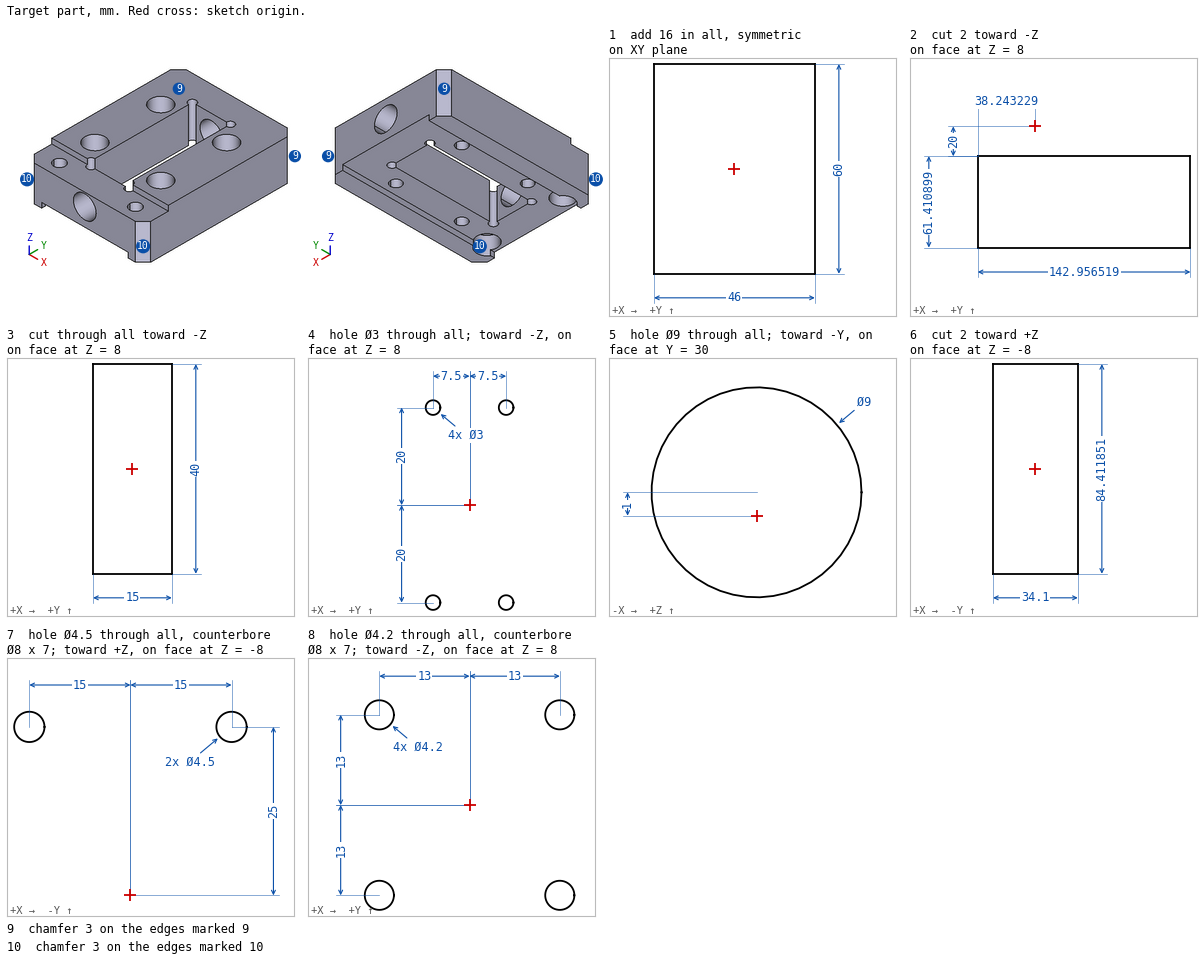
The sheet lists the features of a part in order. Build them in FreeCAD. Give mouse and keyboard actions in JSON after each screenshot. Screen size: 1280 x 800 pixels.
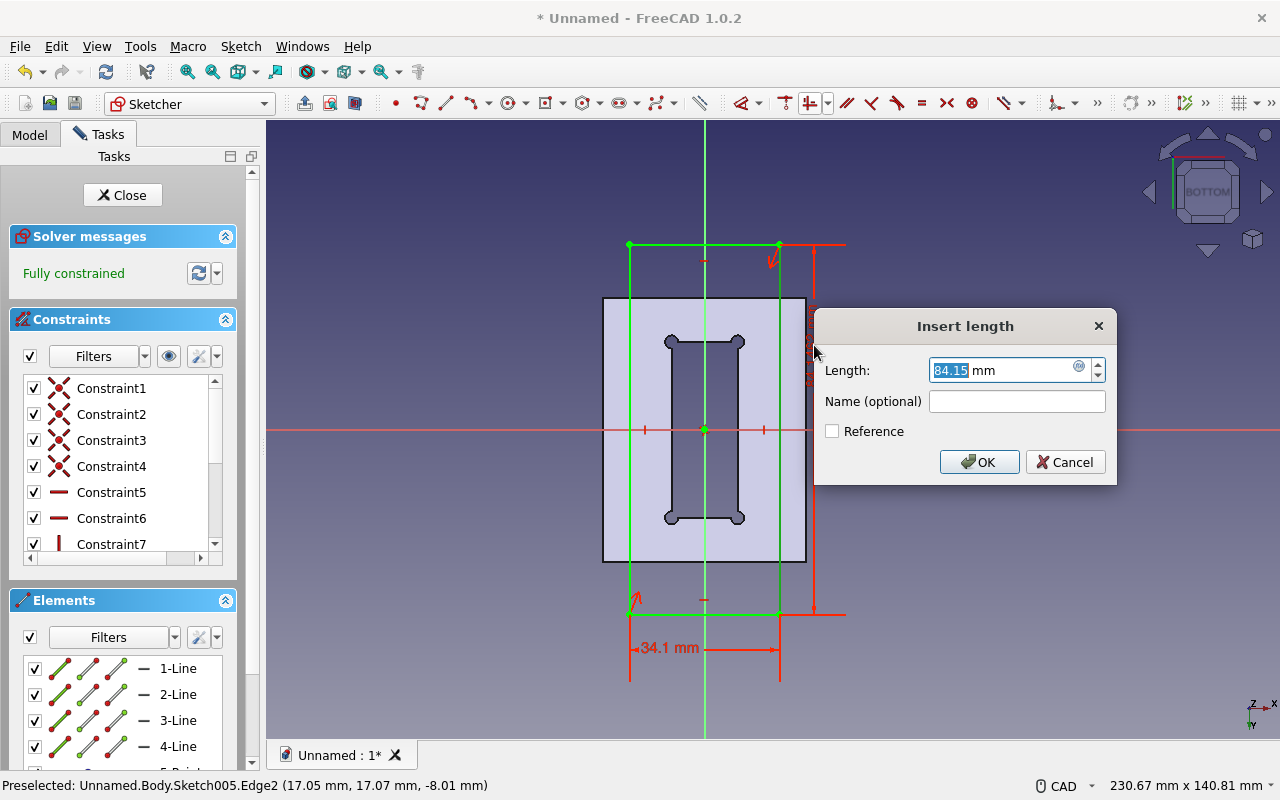
{"action": "type", "text": "84.411851"}
{"action": "key", "text": "Return"}
{"action": "key", "text": "Escape"}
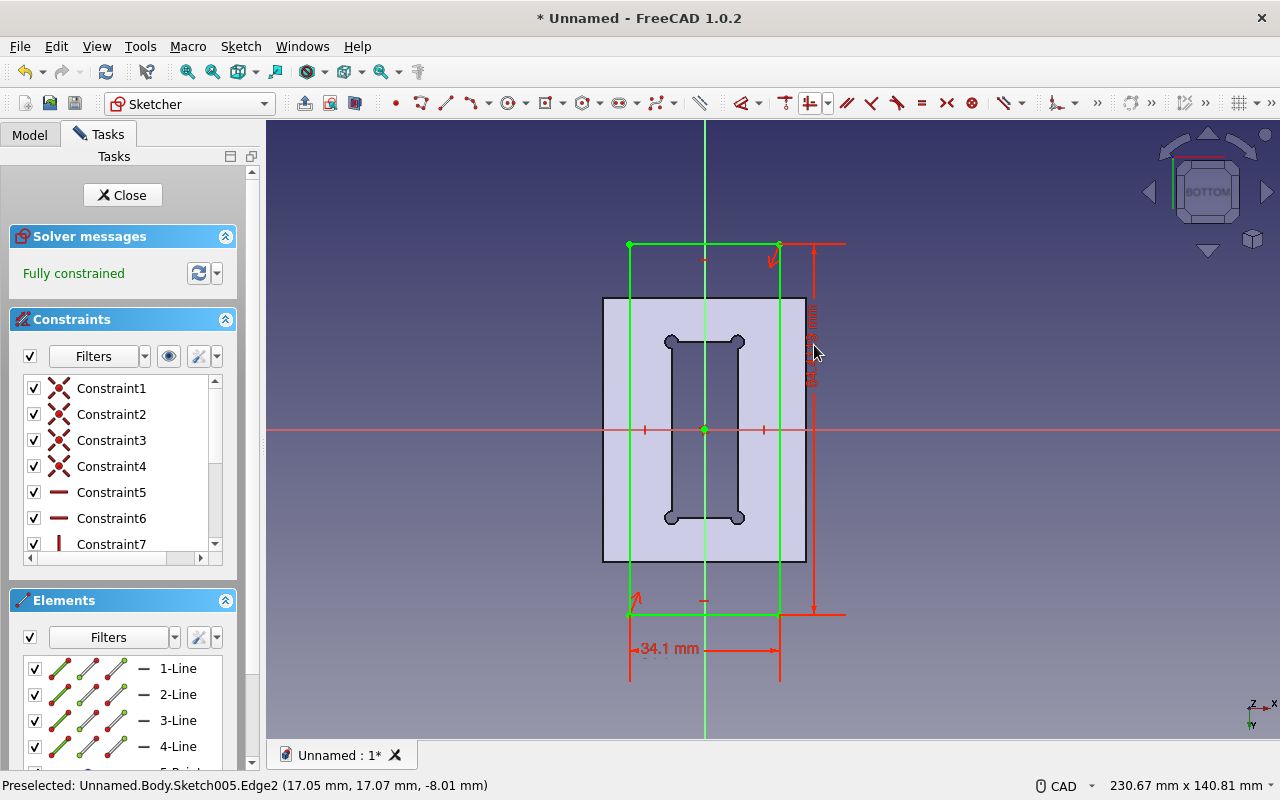
{"action": "left_click", "coordinate": [123, 195]}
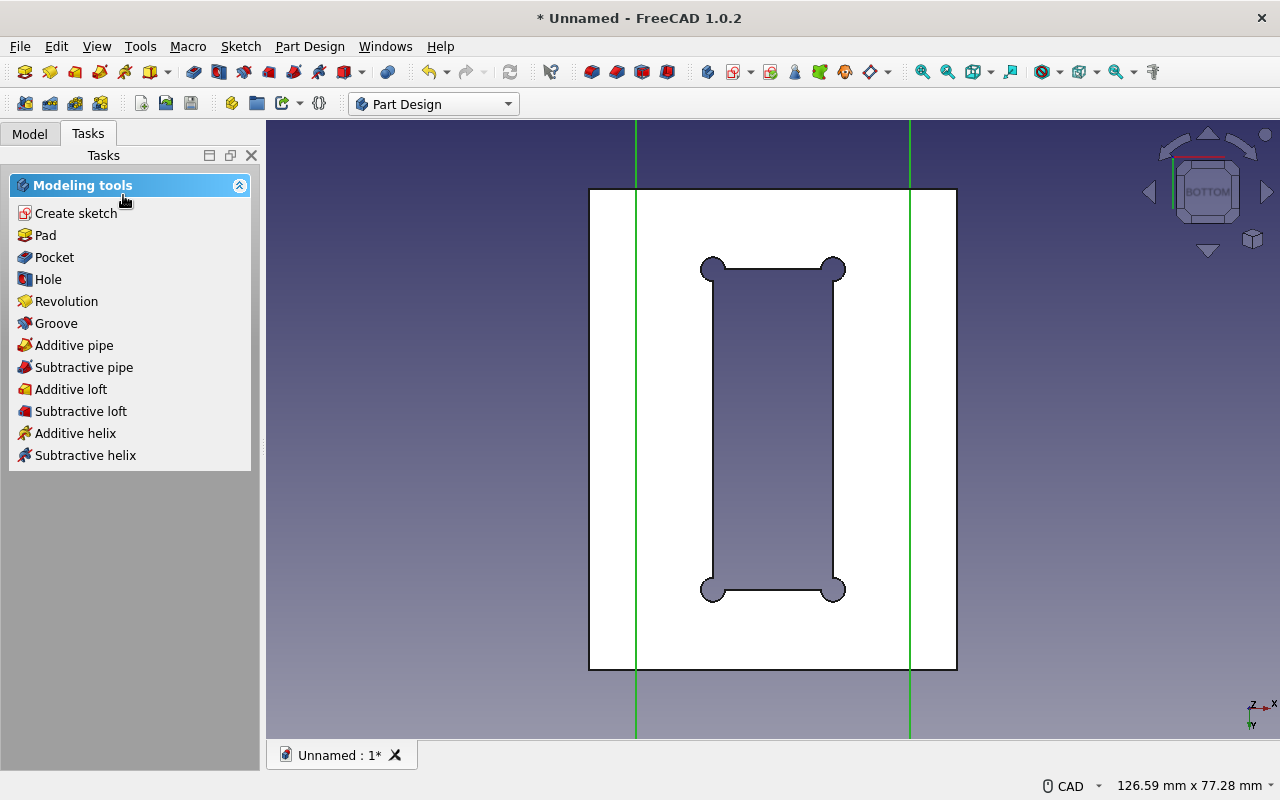
{"action": "left_click", "coordinate": [194, 72]}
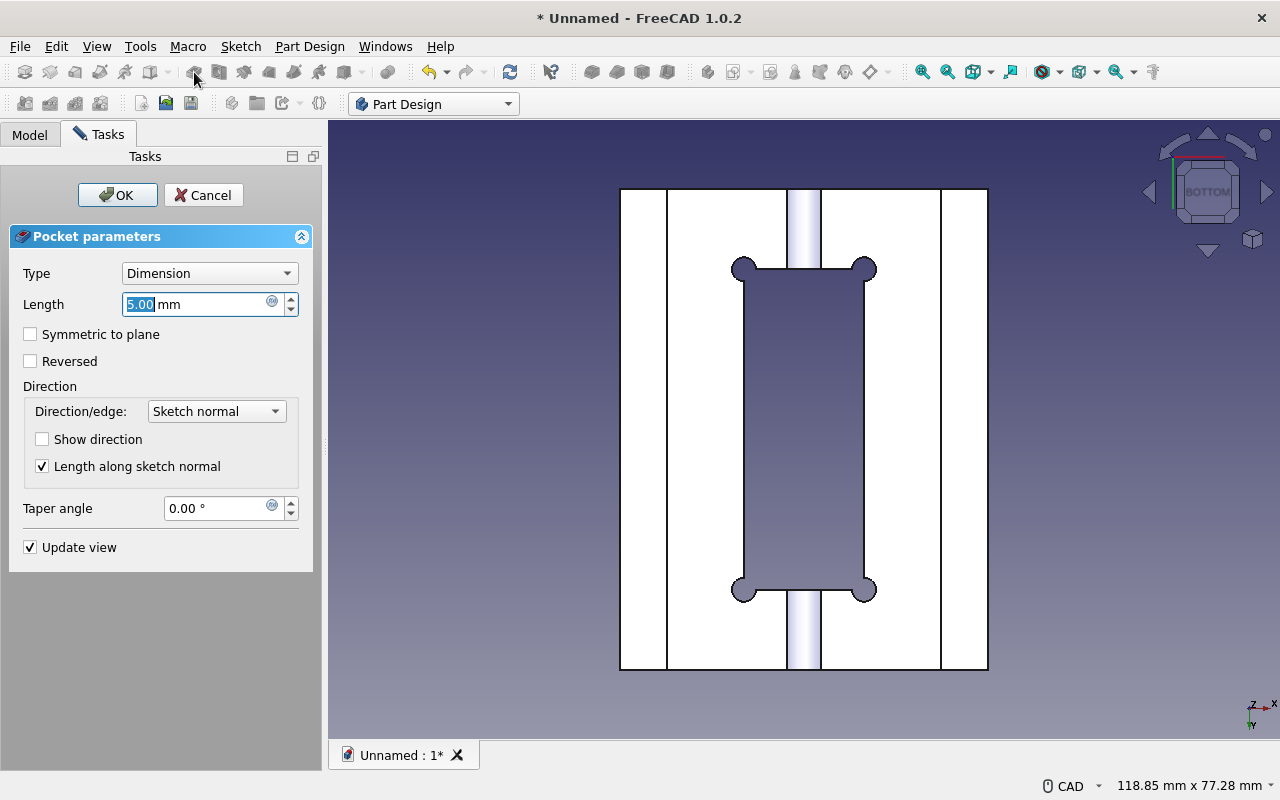
{"action": "type", "text": "2"}
{"action": "key", "text": "Tab"}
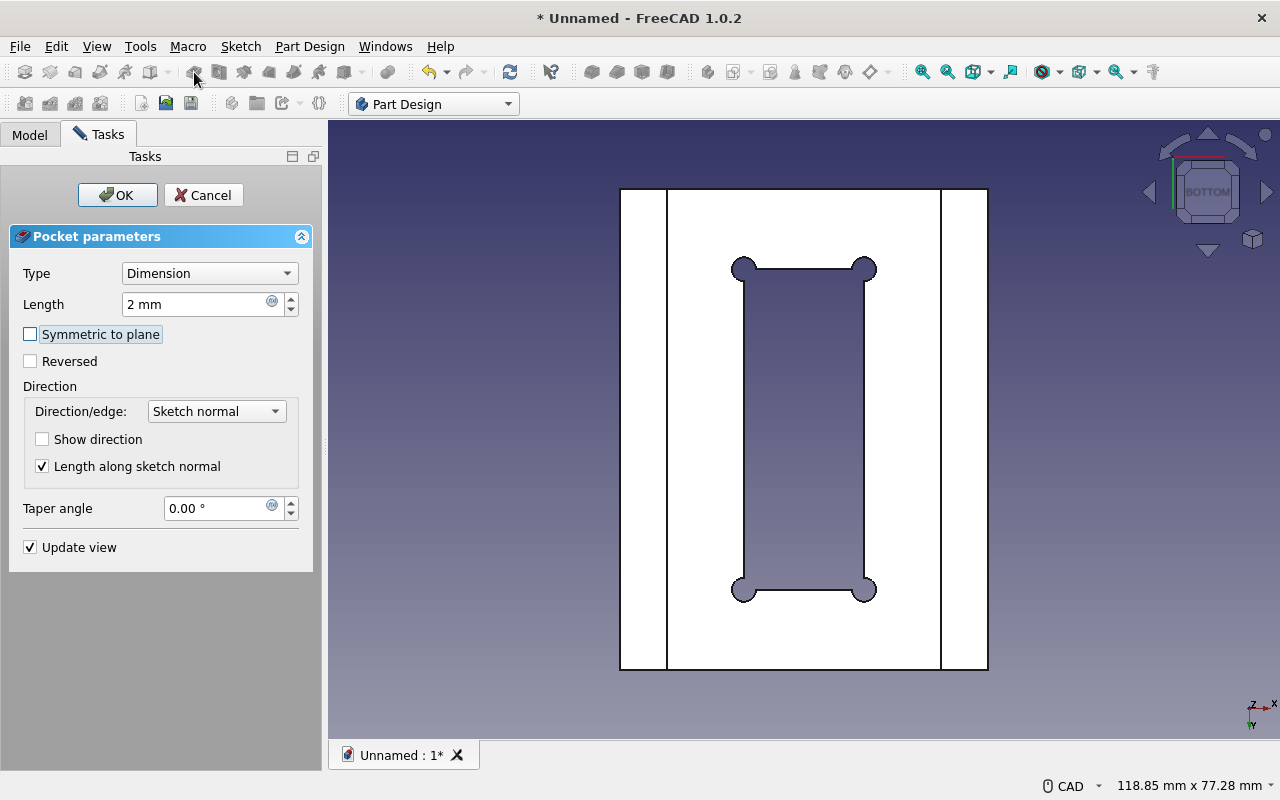
{"action": "left_click", "coordinate": [118, 195]}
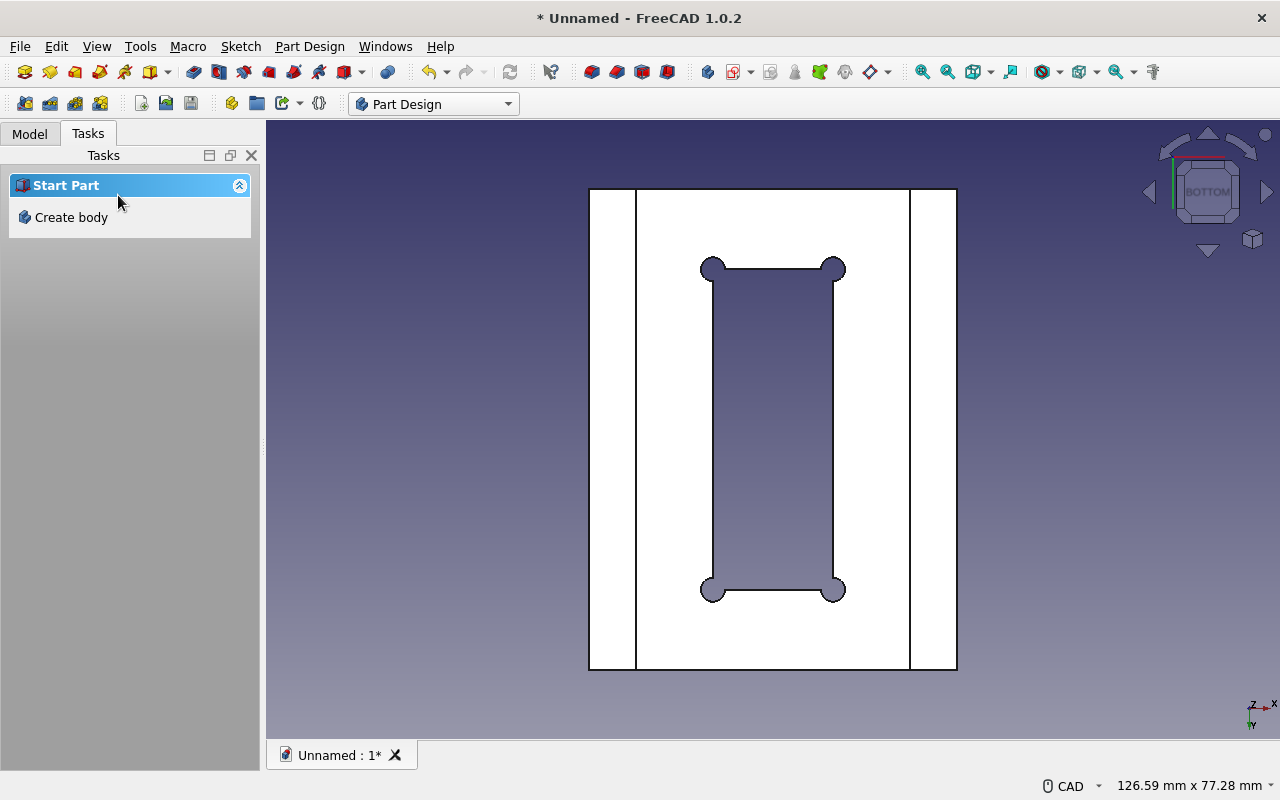
{"action": "left_click", "coordinate": [613, 634]}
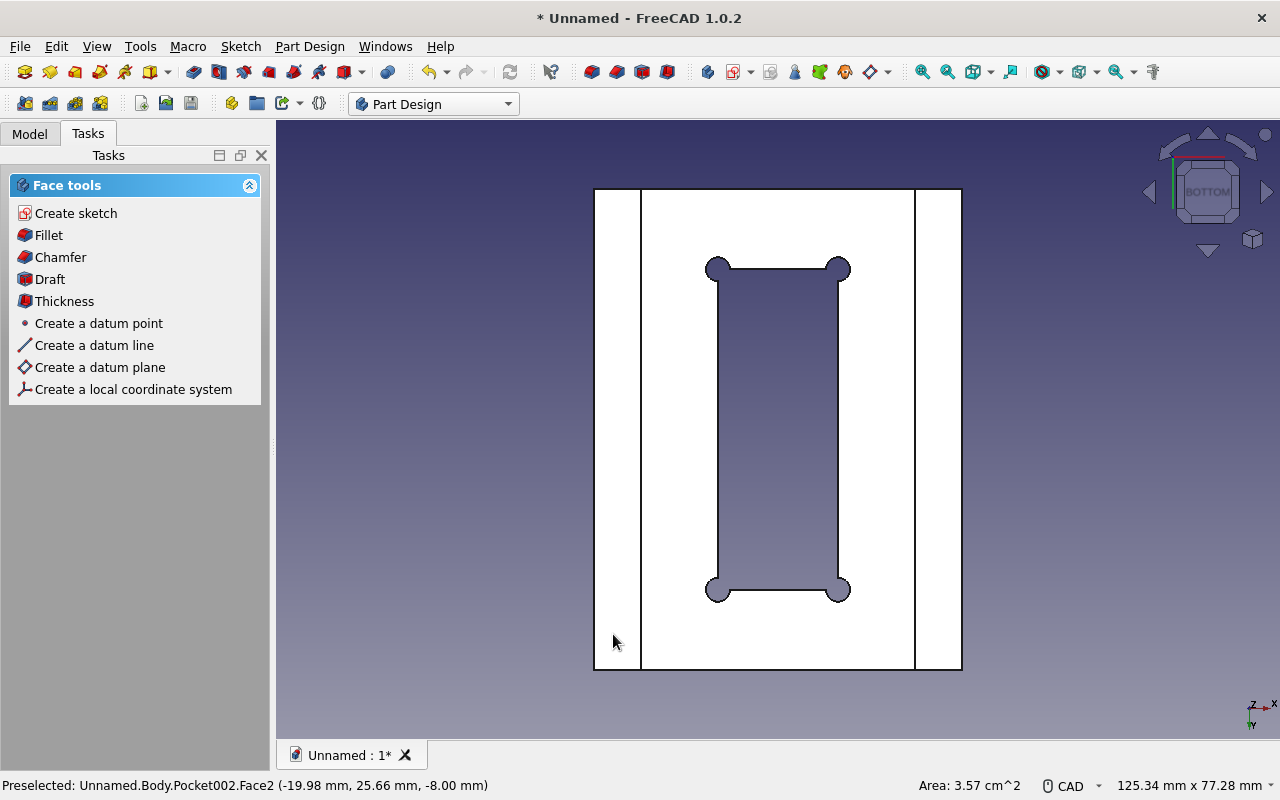
{"action": "left_click", "coordinate": [732, 72]}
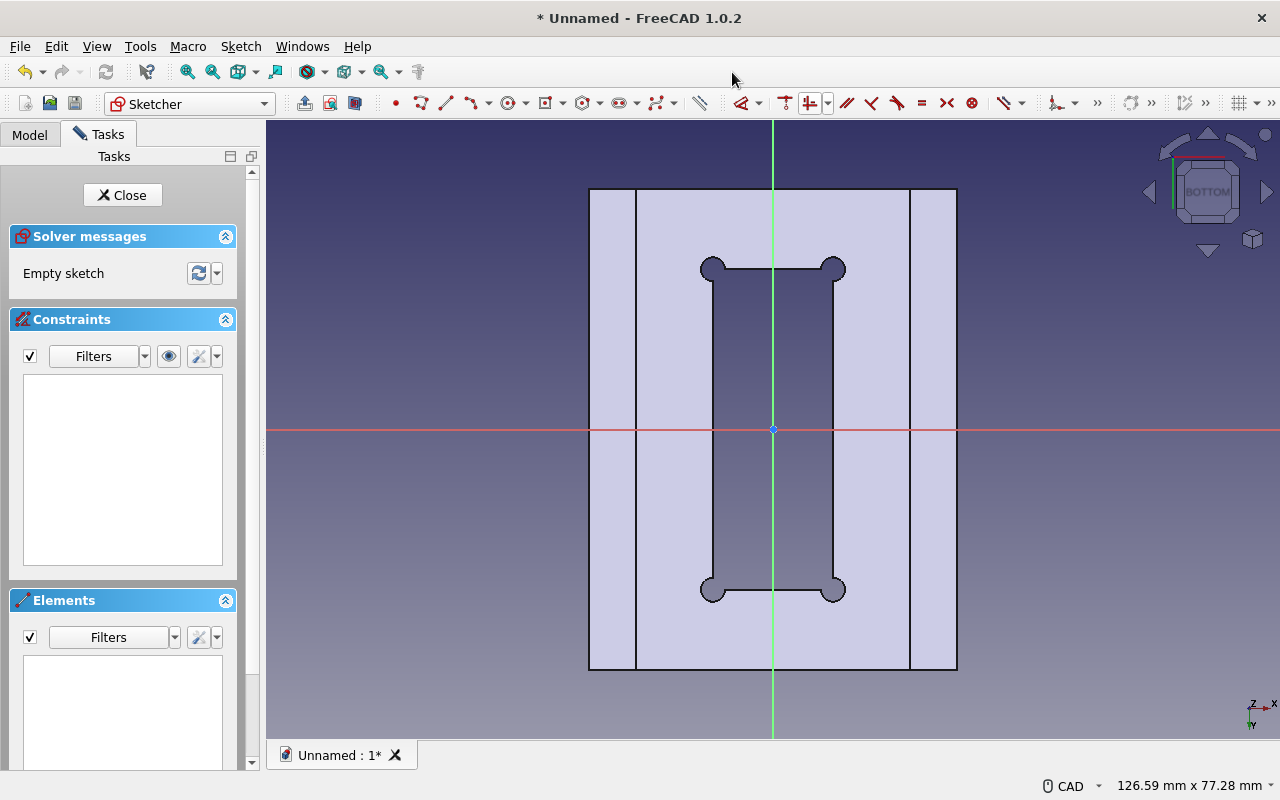
{"action": "scroll", "coordinate": [856, 188], "scroll_direction": "up", "scroll_amount": 3}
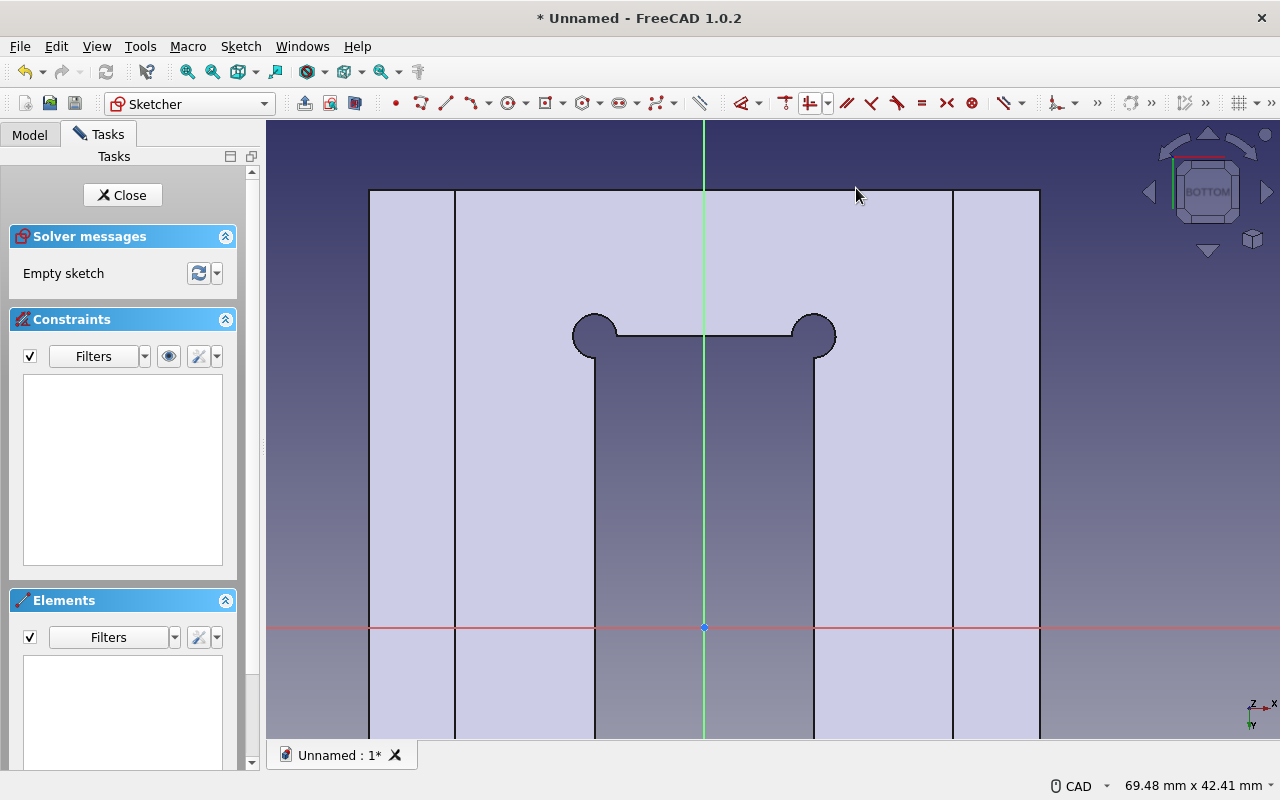
{"action": "left_click", "coordinate": [508, 104]}